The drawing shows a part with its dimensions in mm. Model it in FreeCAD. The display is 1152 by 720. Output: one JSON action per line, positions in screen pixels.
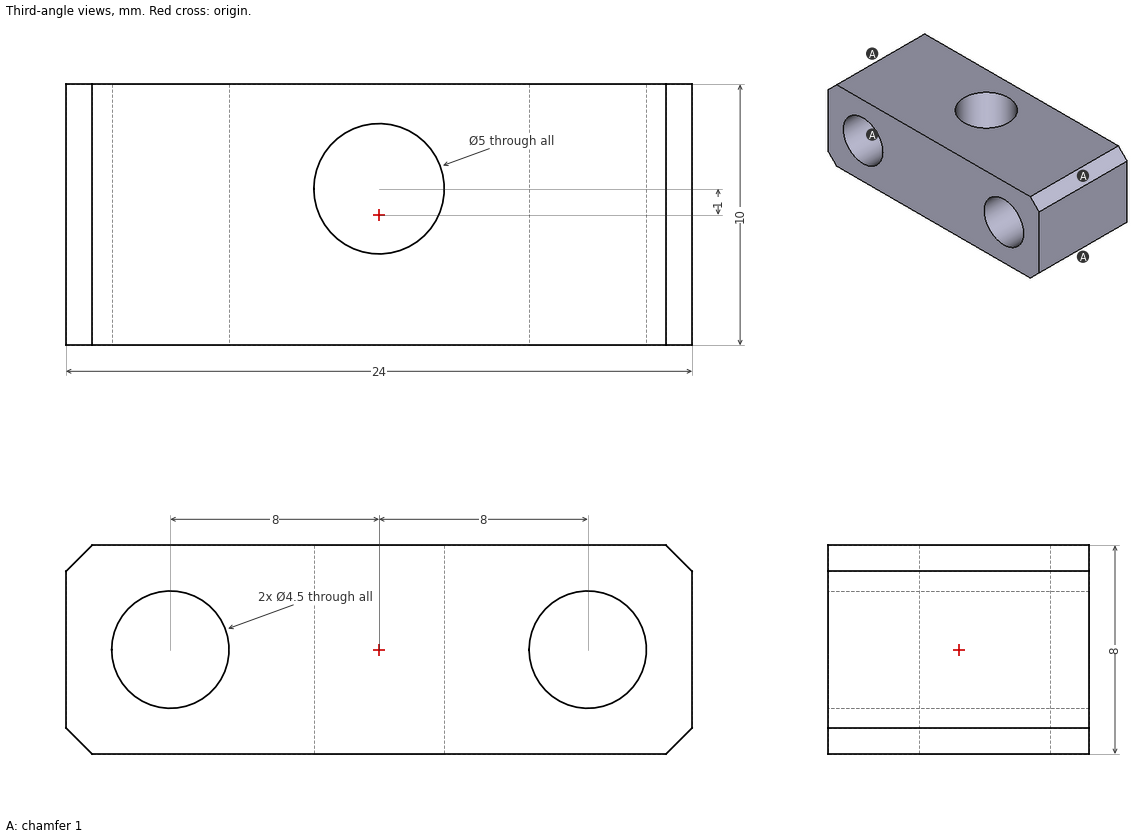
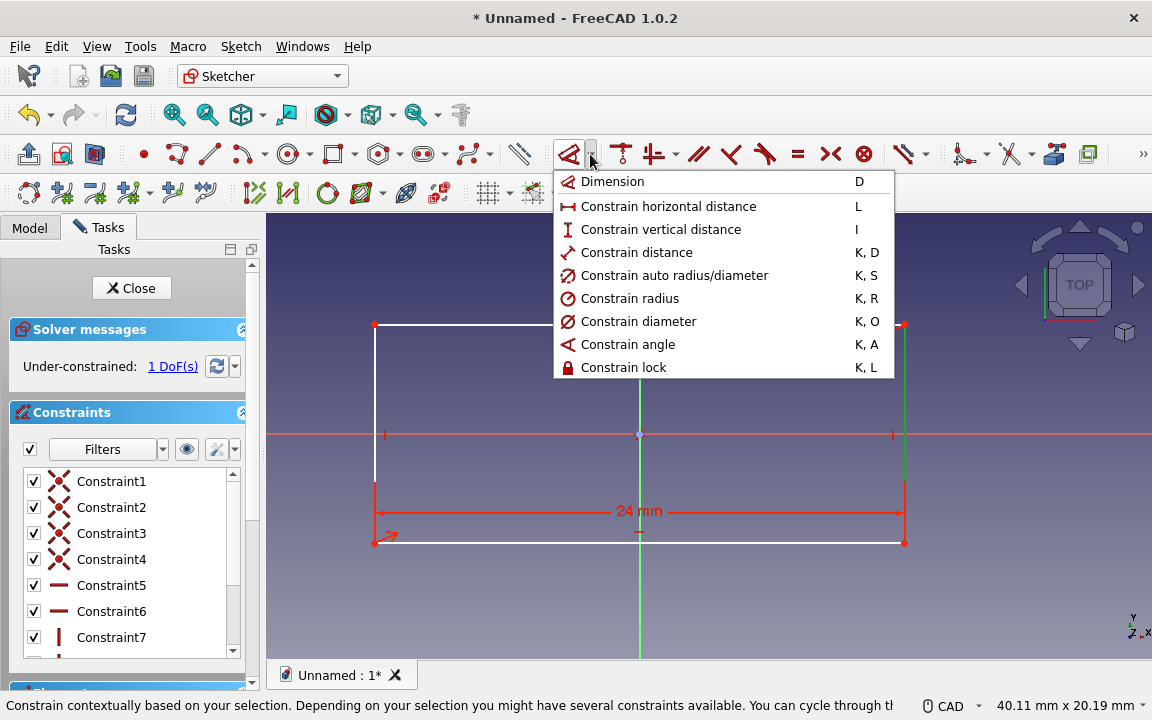
{"action": "left_click", "coordinate": [724, 230]}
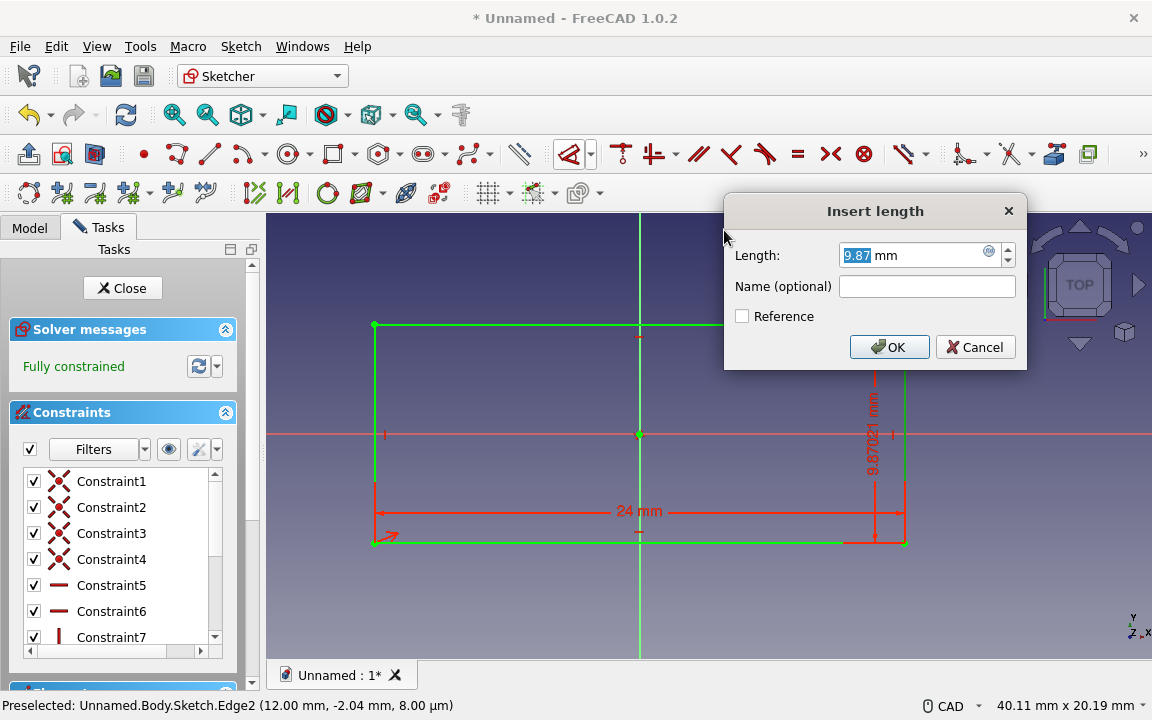
{"action": "type", "text": "10"}
{"action": "key", "text": "Return"}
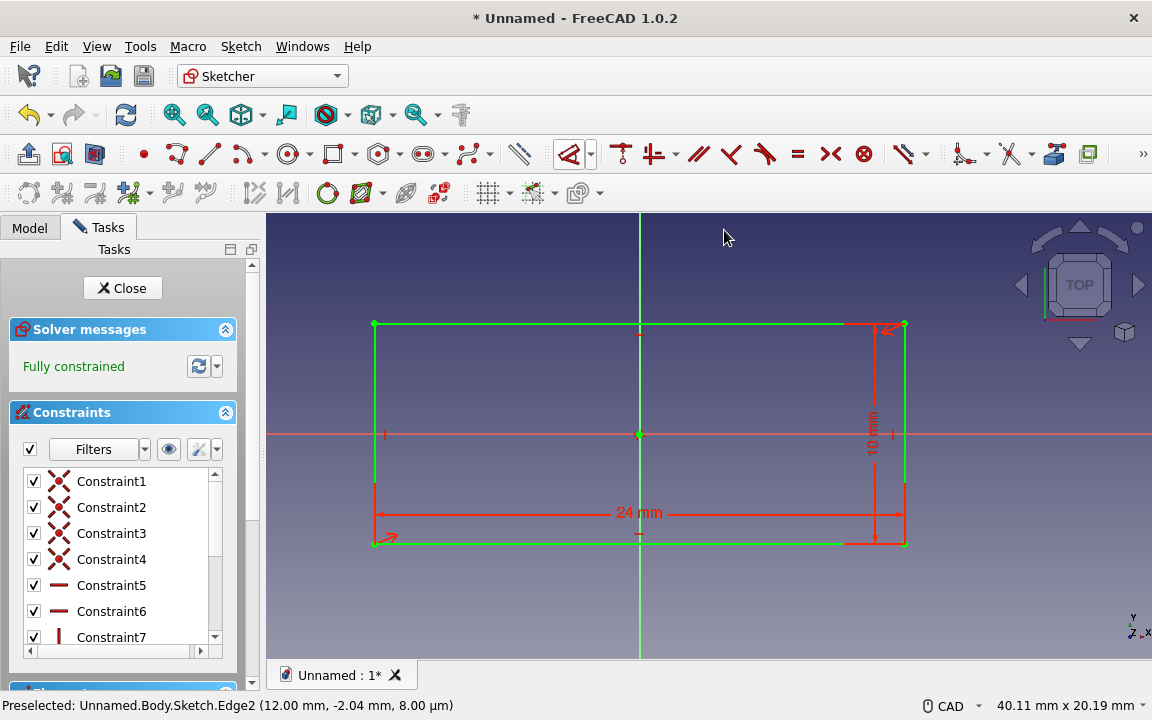
{"action": "left_click", "coordinate": [123, 288]}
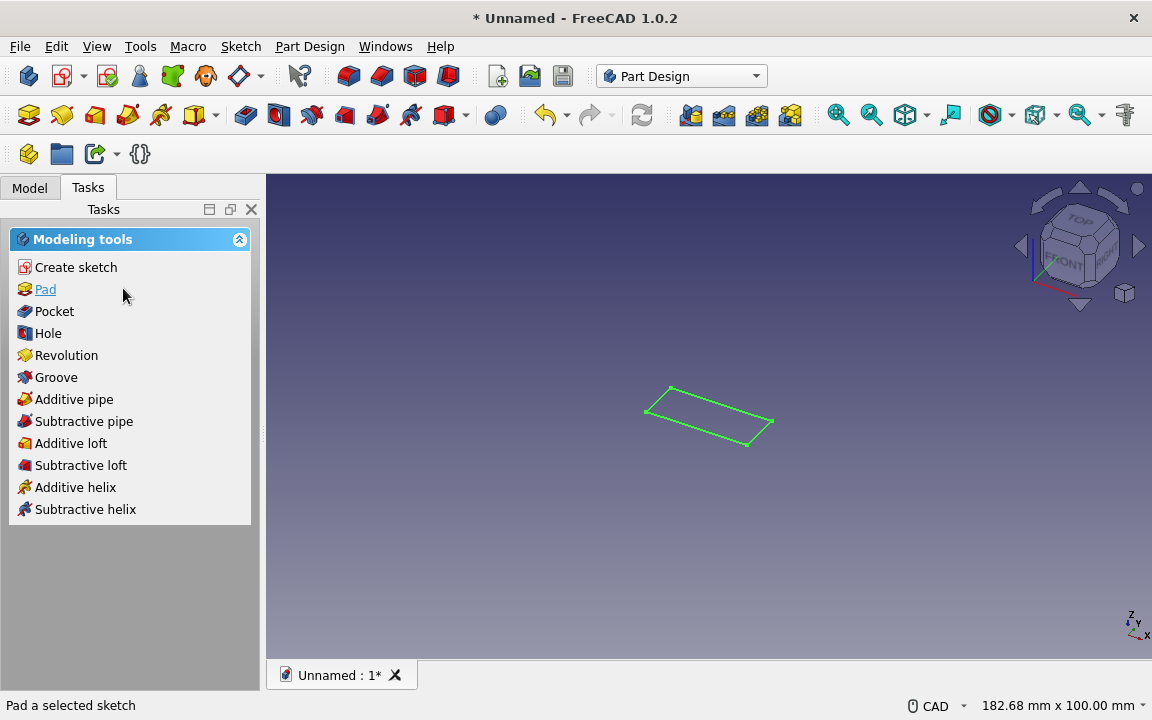
{"action": "left_click", "coordinate": [29, 116]}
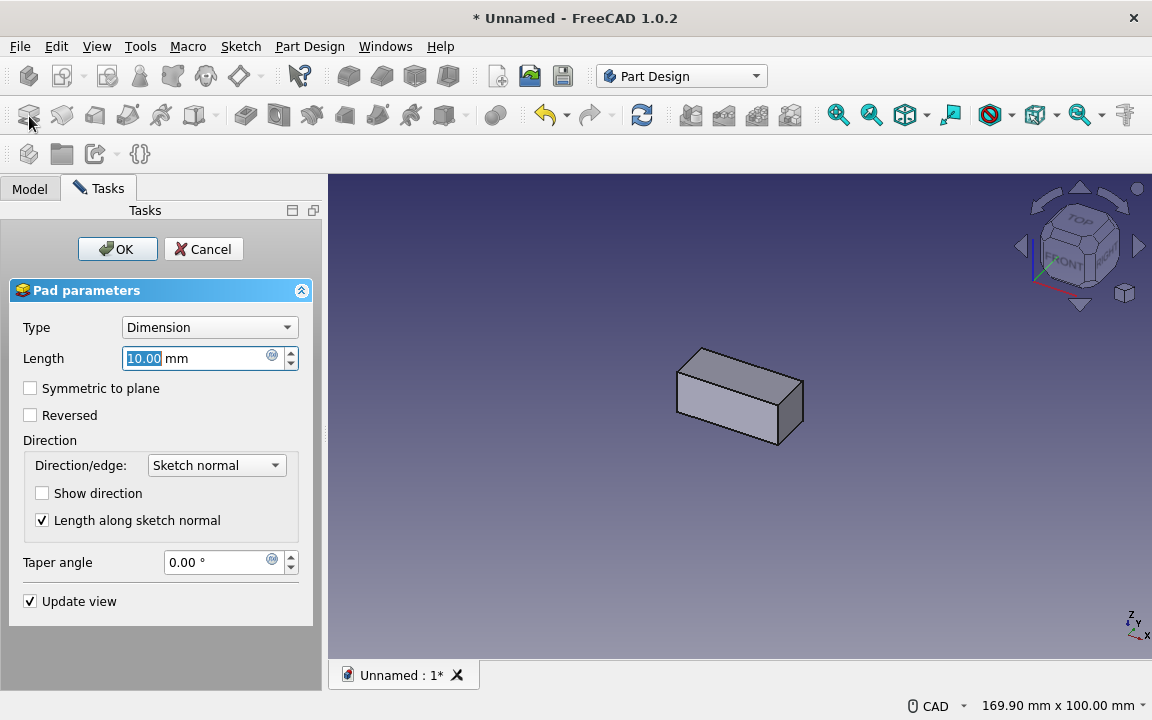
{"action": "type", "text": "8"}
{"action": "key", "text": "Tab"}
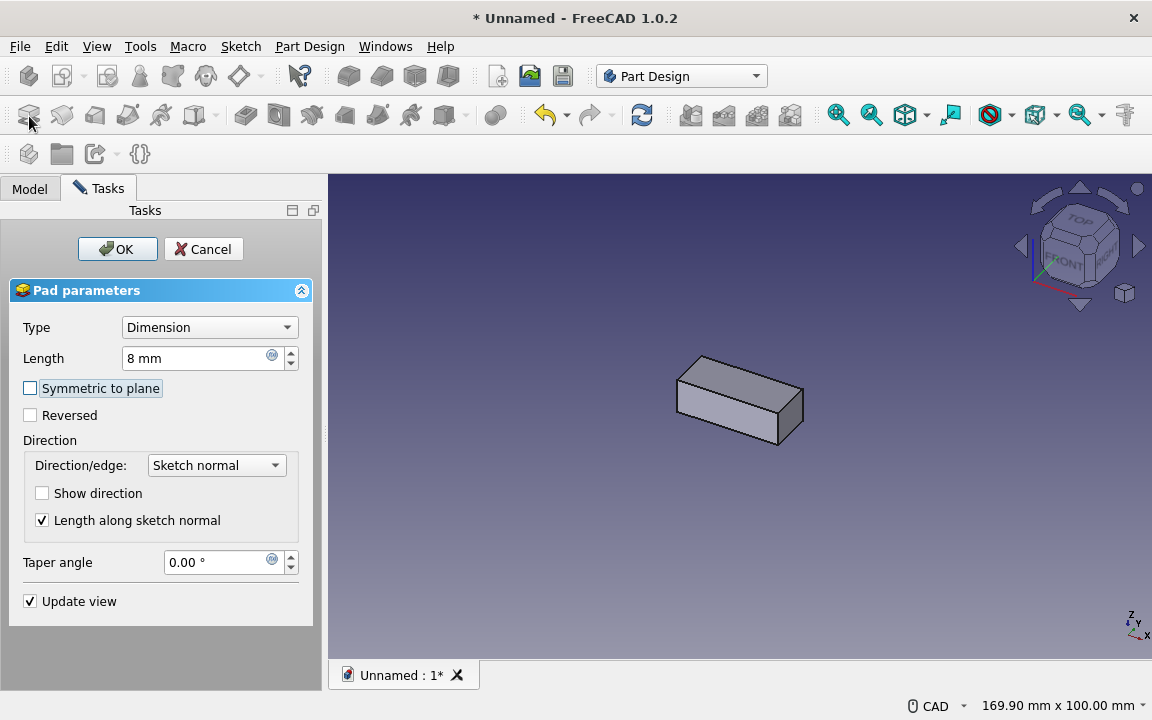
{"action": "left_click", "coordinate": [31, 388]}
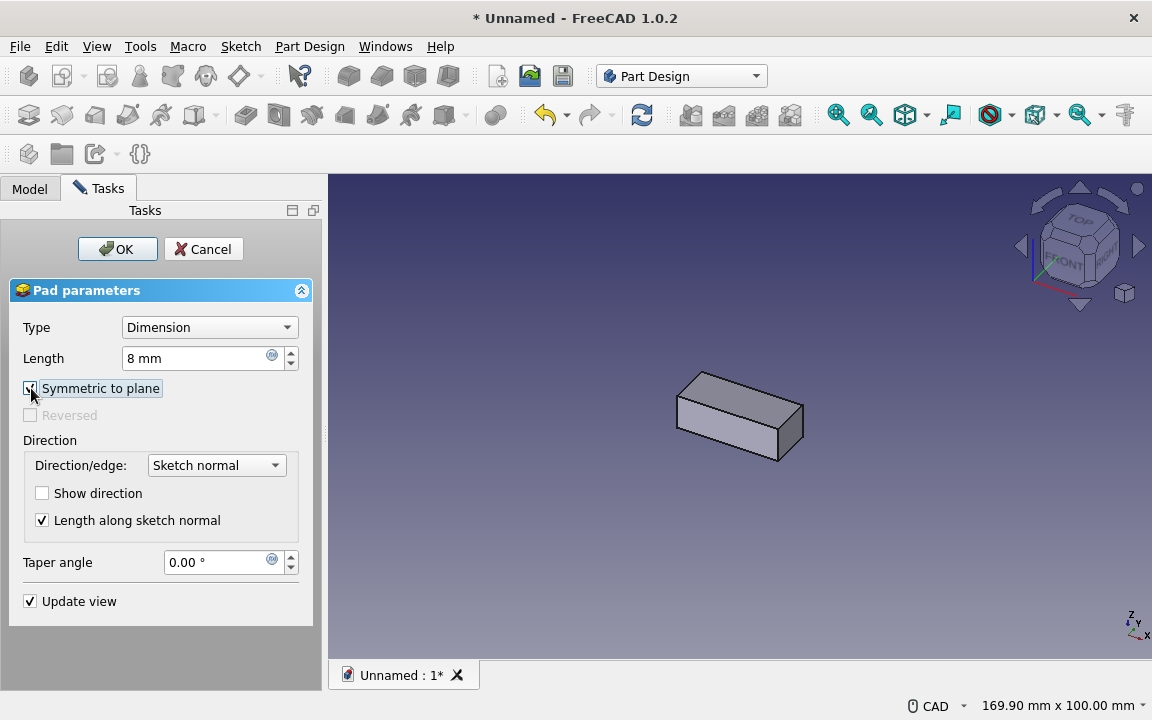
{"action": "left_click", "coordinate": [118, 249]}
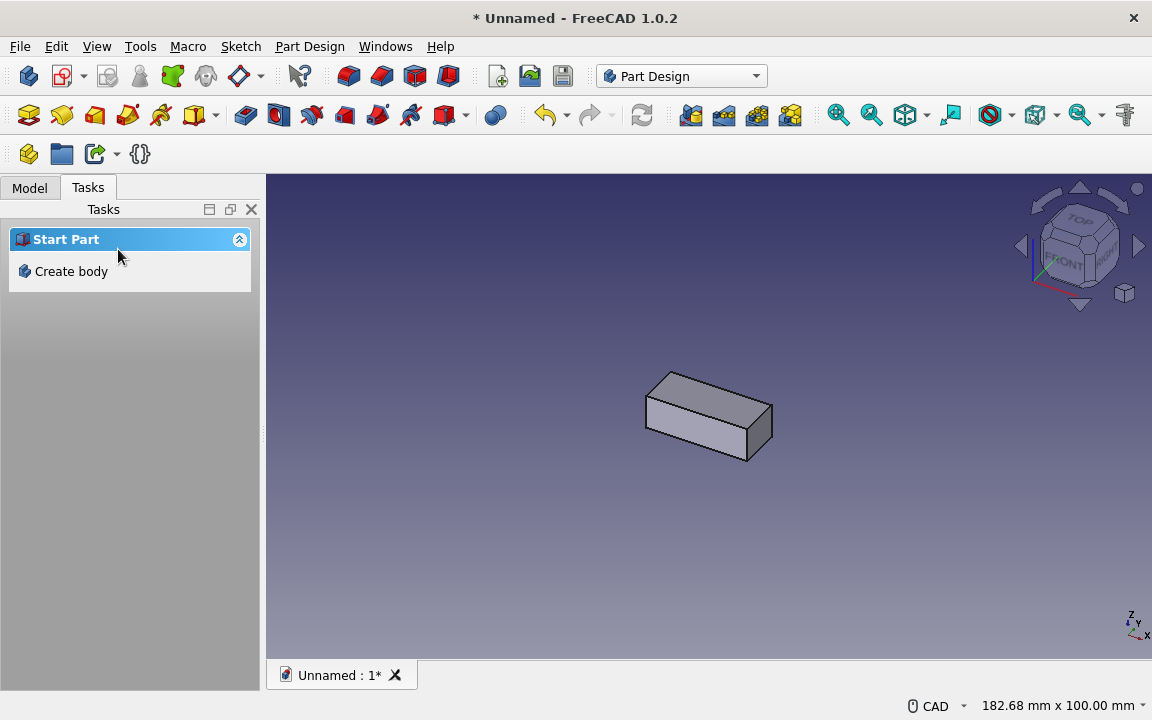
{"action": "left_click", "coordinate": [839, 116]}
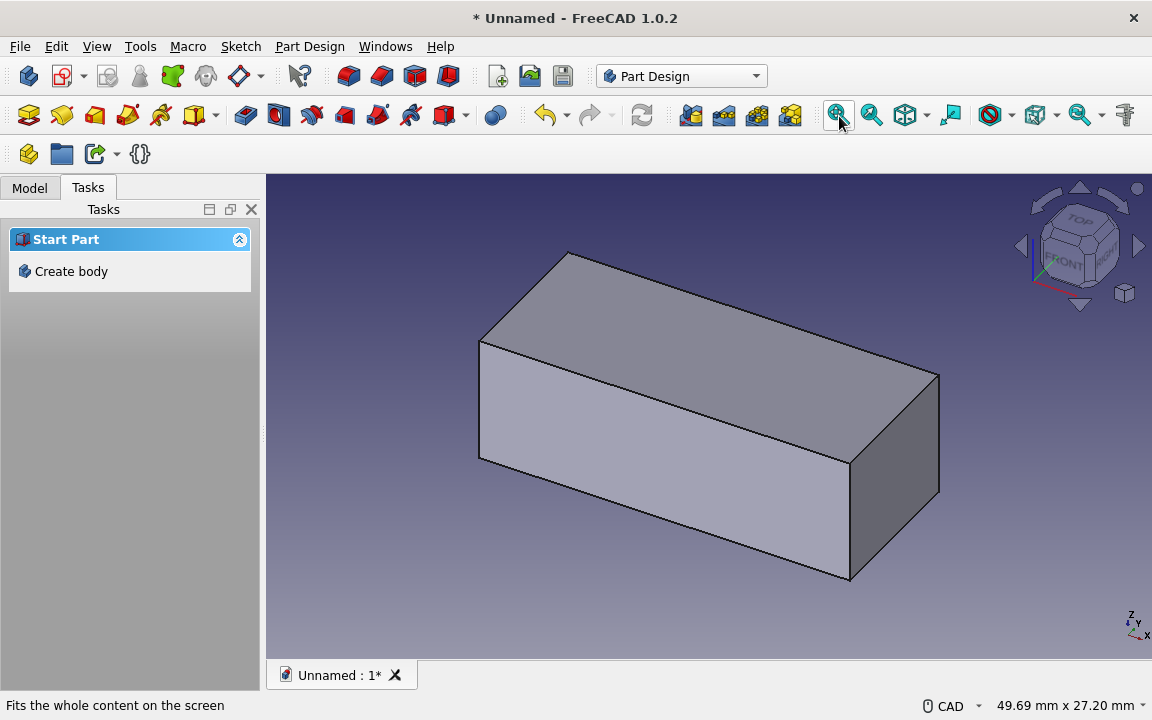
{"action": "key", "text": "4"}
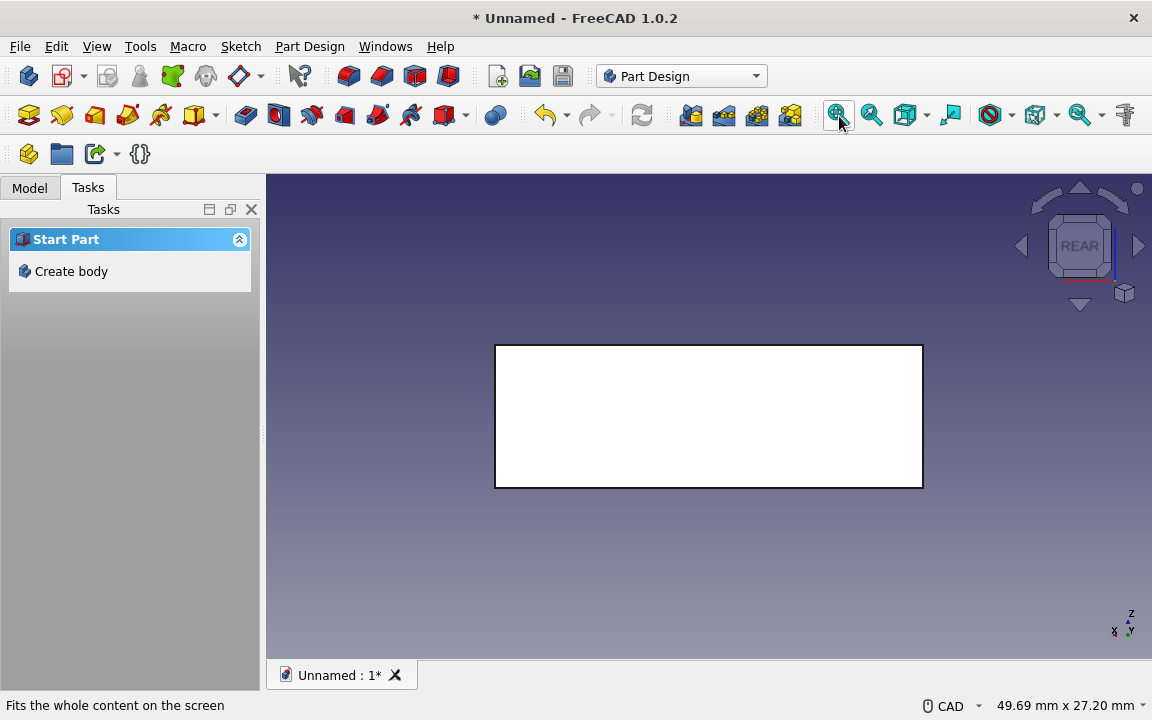
{"action": "left_click", "coordinate": [587, 416]}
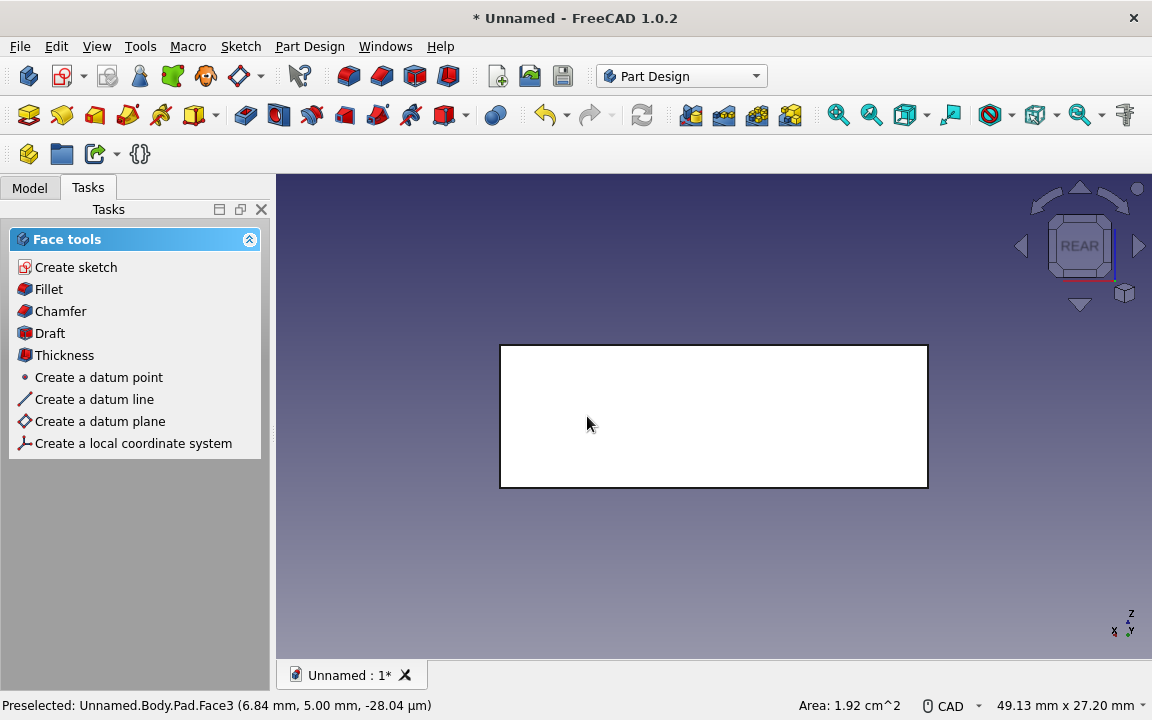
{"action": "left_click", "coordinate": [62, 76]}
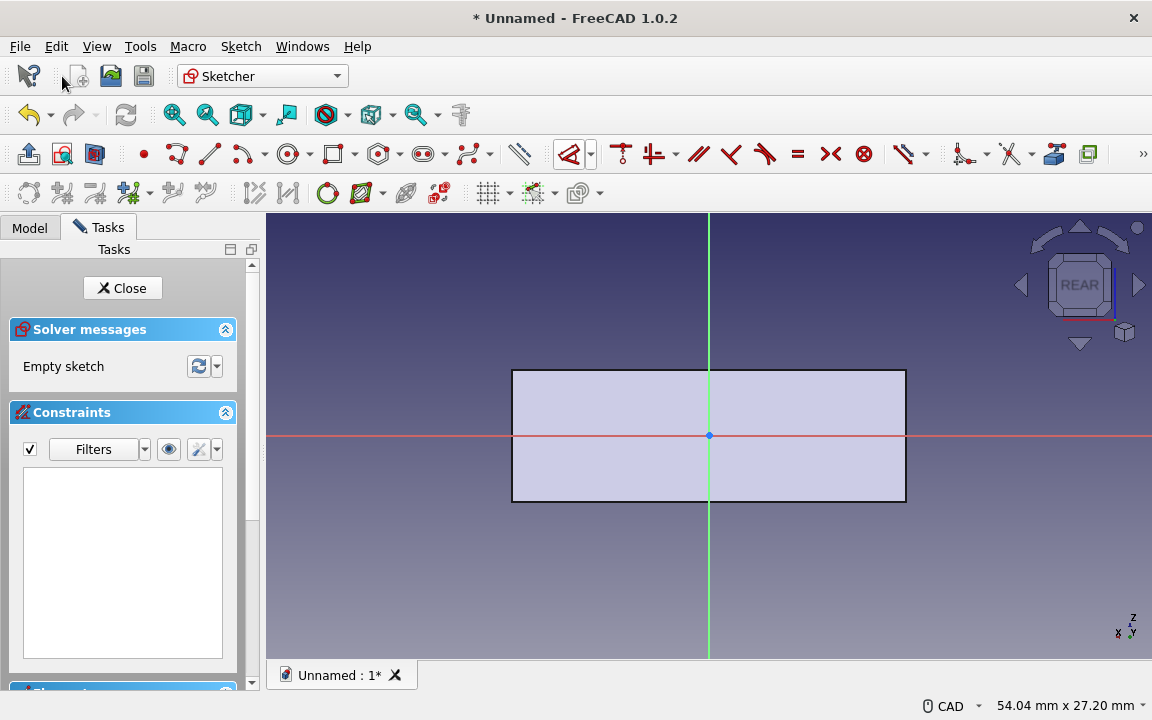
{"action": "scroll", "coordinate": [848, 436], "scroll_direction": "up", "scroll_amount": 2}